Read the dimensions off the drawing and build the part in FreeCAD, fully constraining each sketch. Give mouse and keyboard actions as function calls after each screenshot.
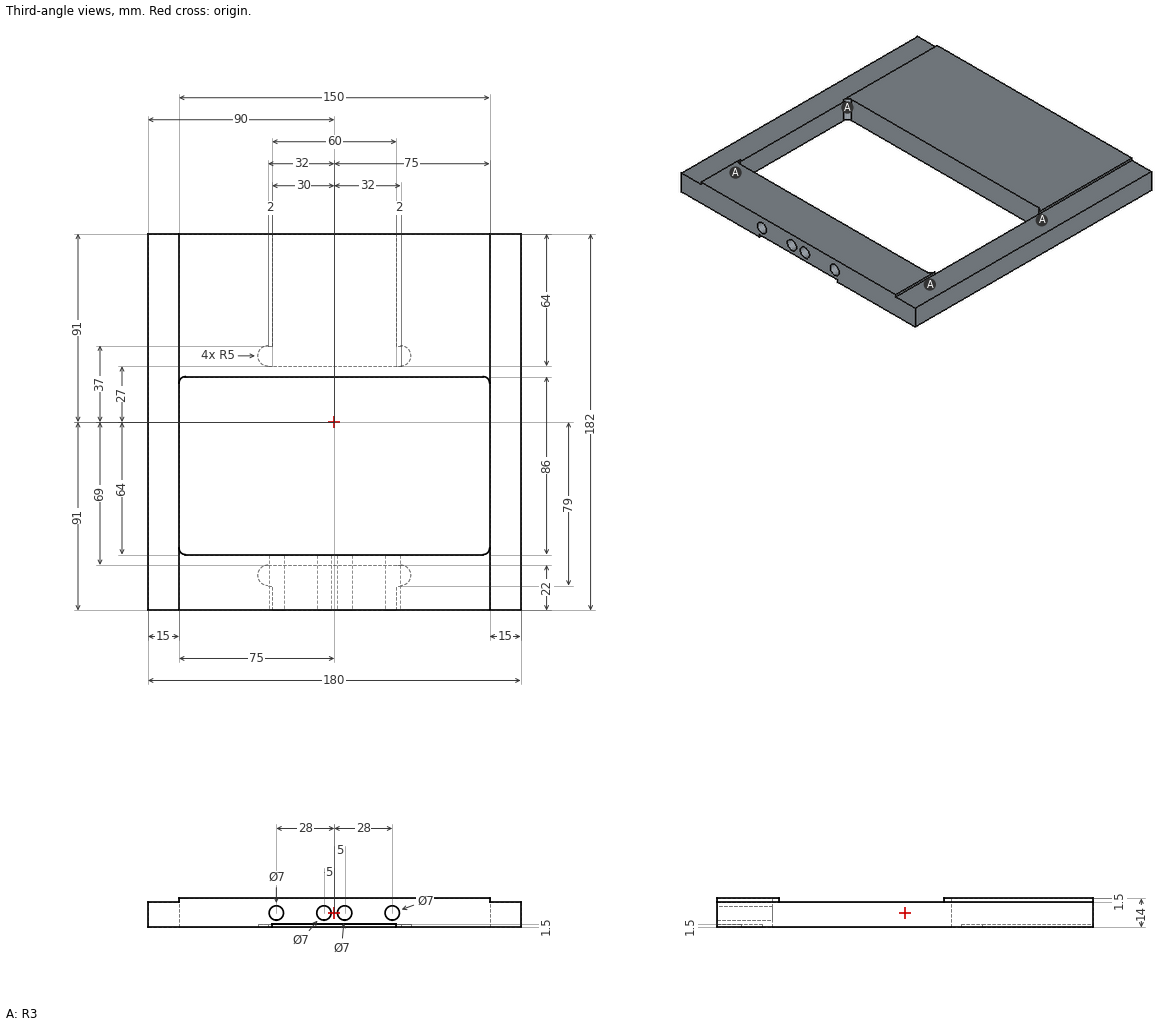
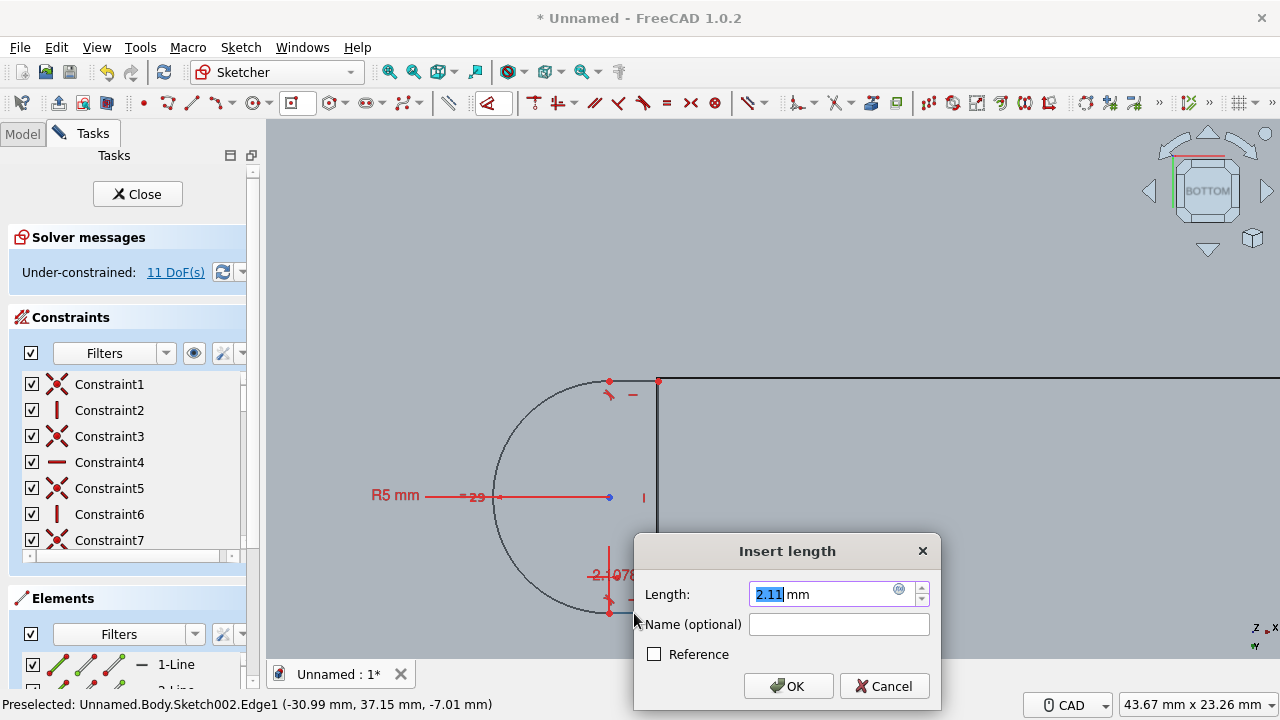
text(2)
key(Return)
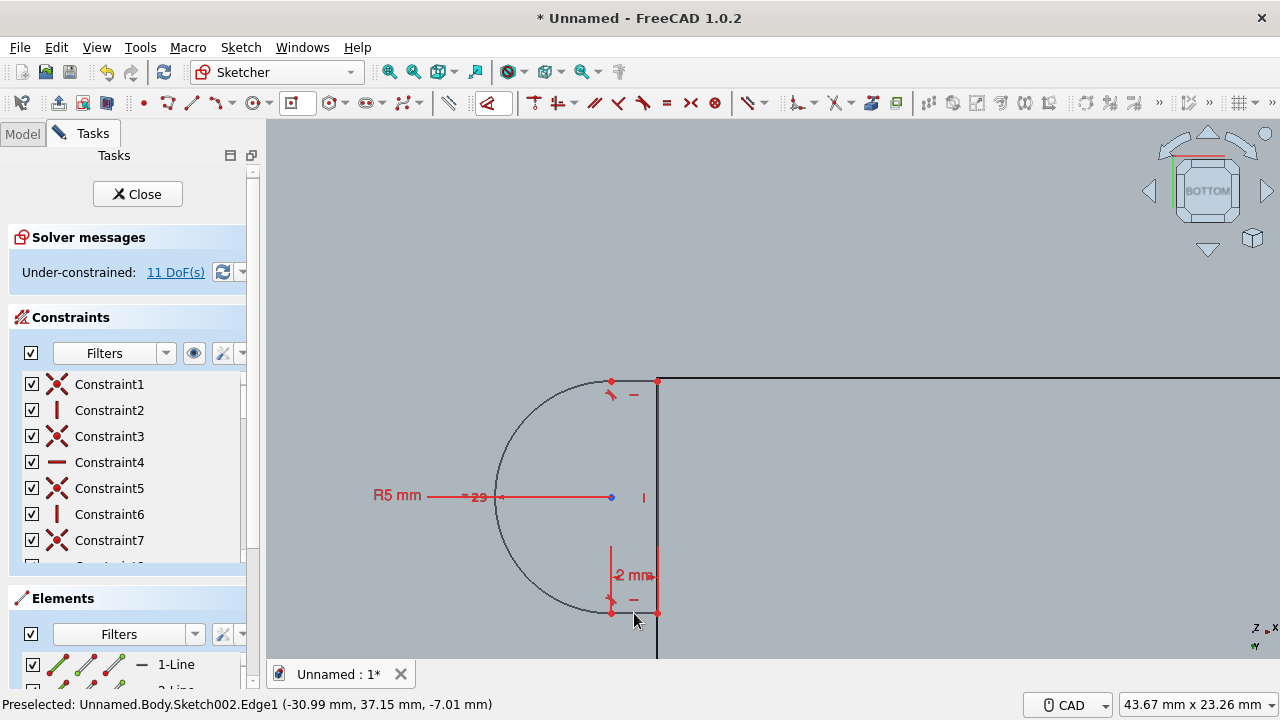
scroll(603, 565, down, 10)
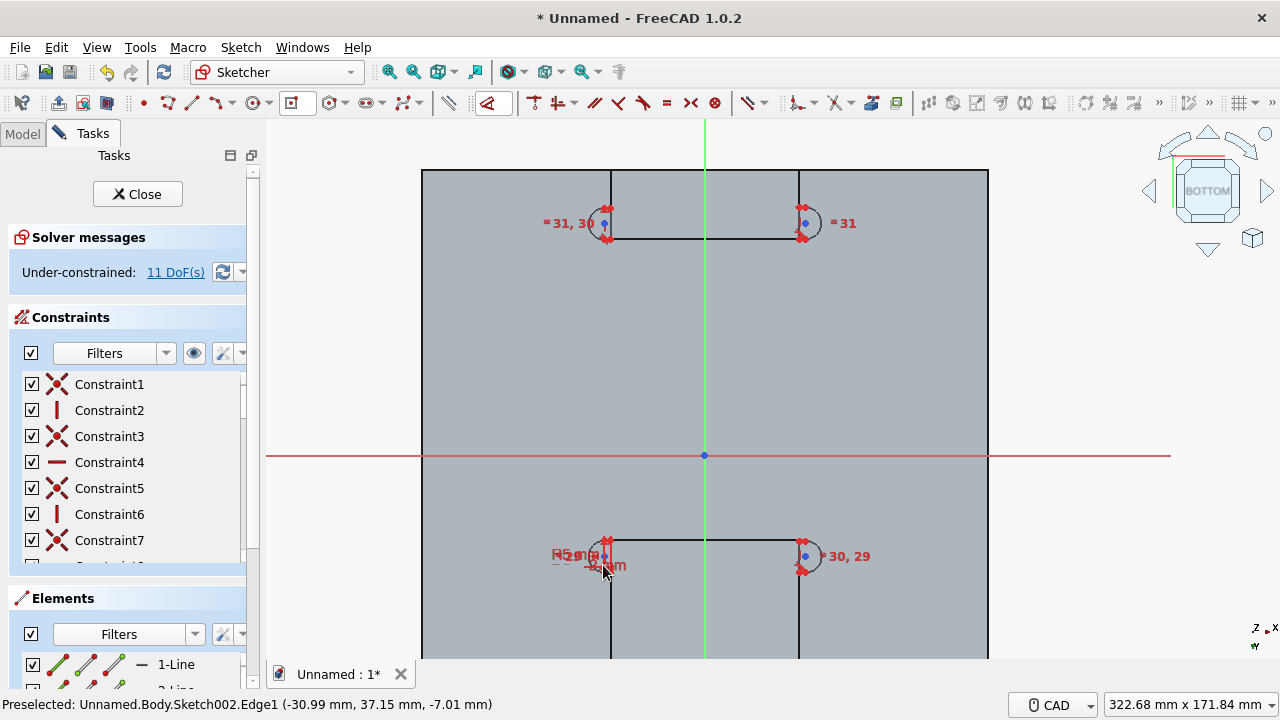
scroll(804, 541, up, 10)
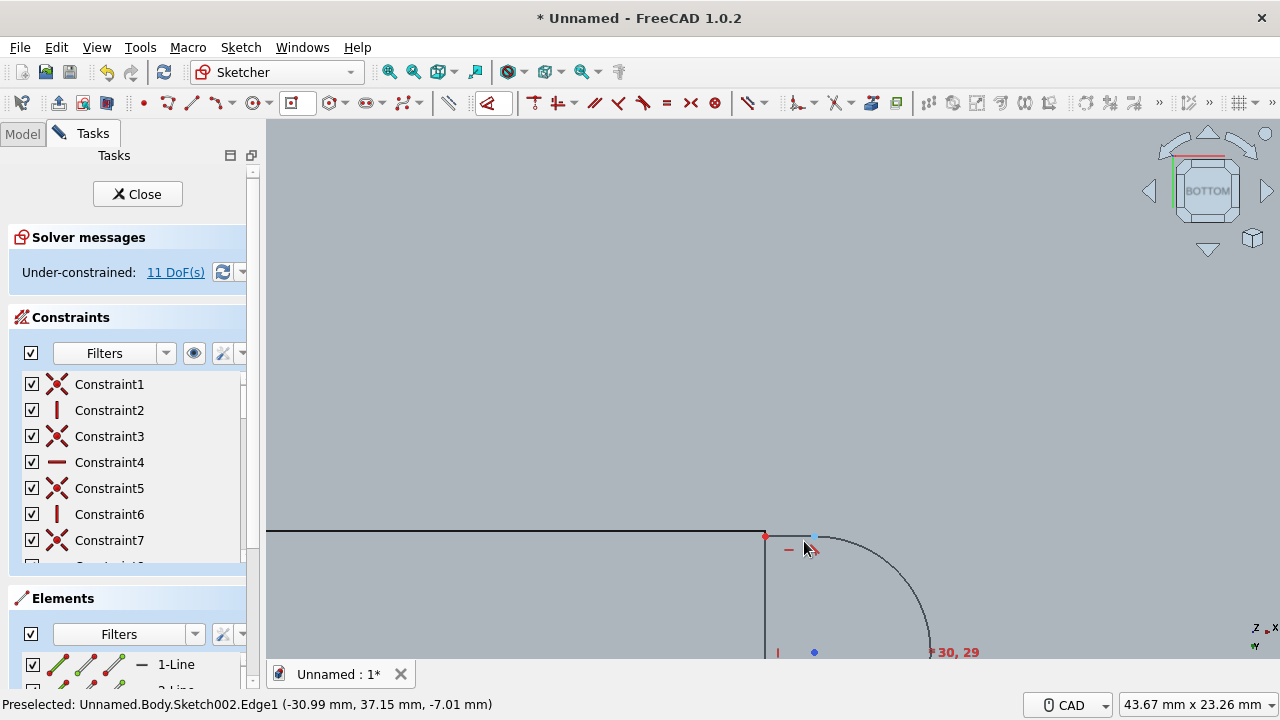
click(800, 536)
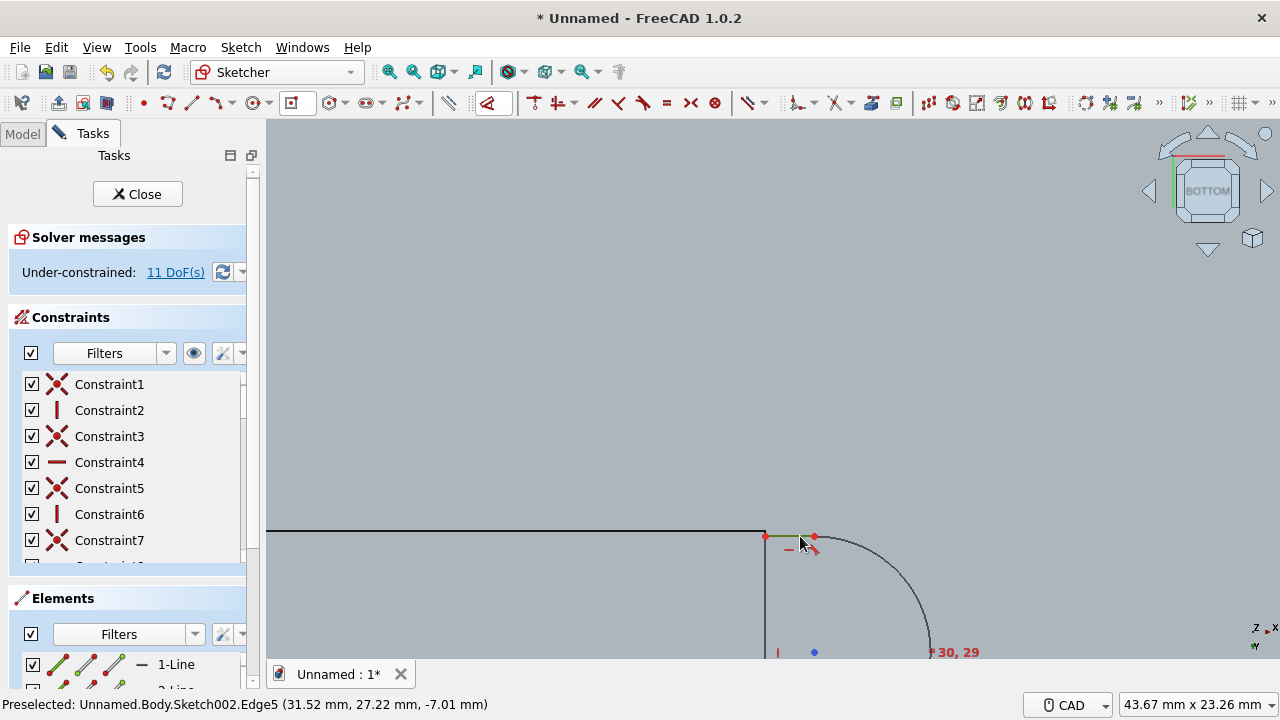
key(l)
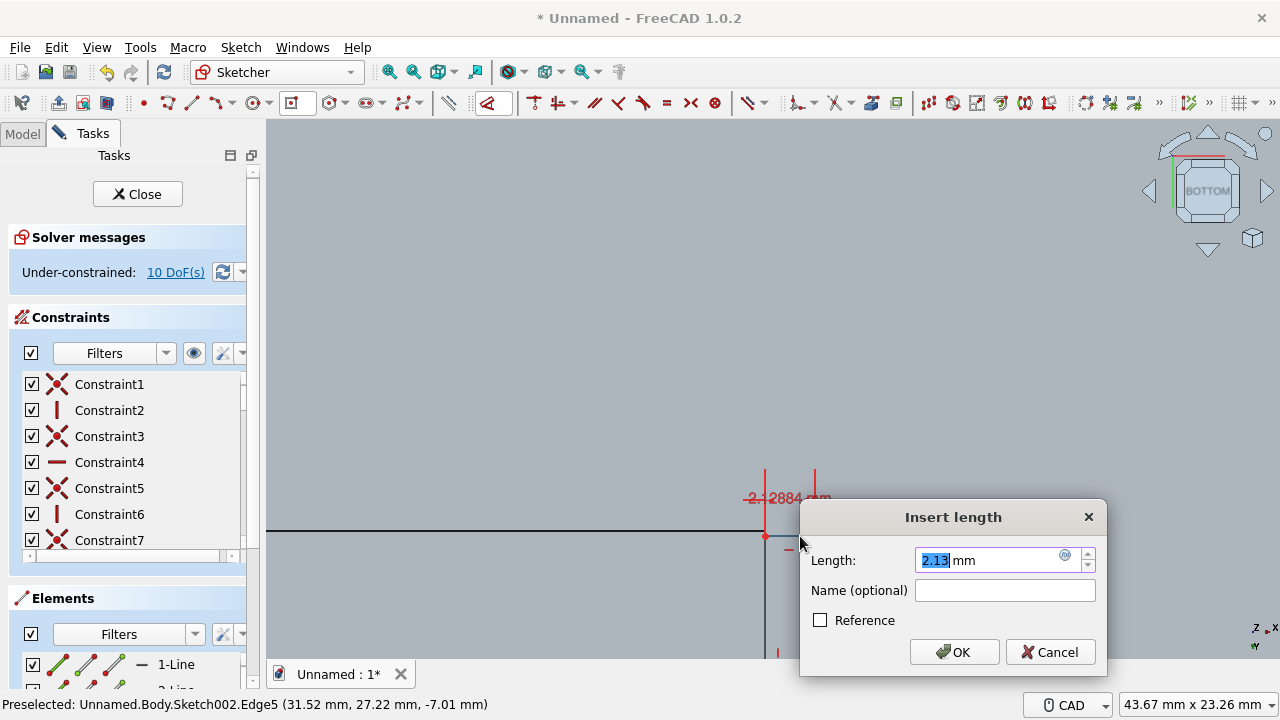
text(2)
key(Return)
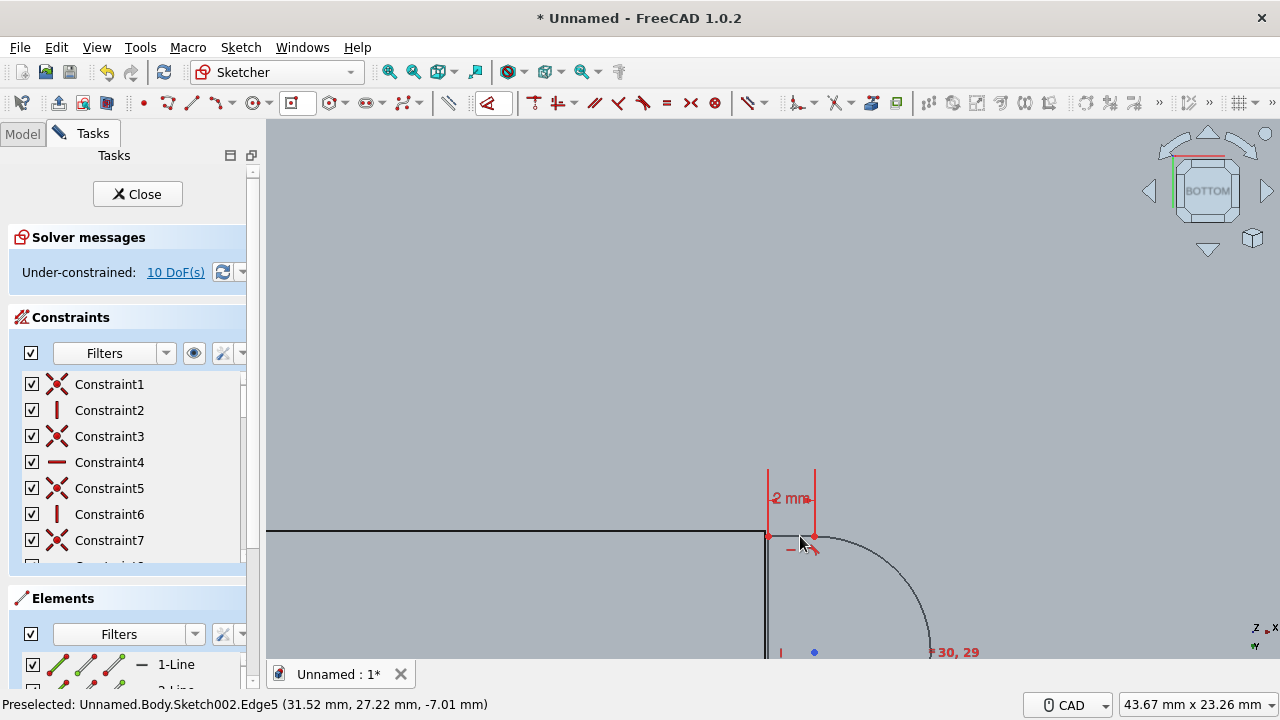
scroll(804, 541, down, 10)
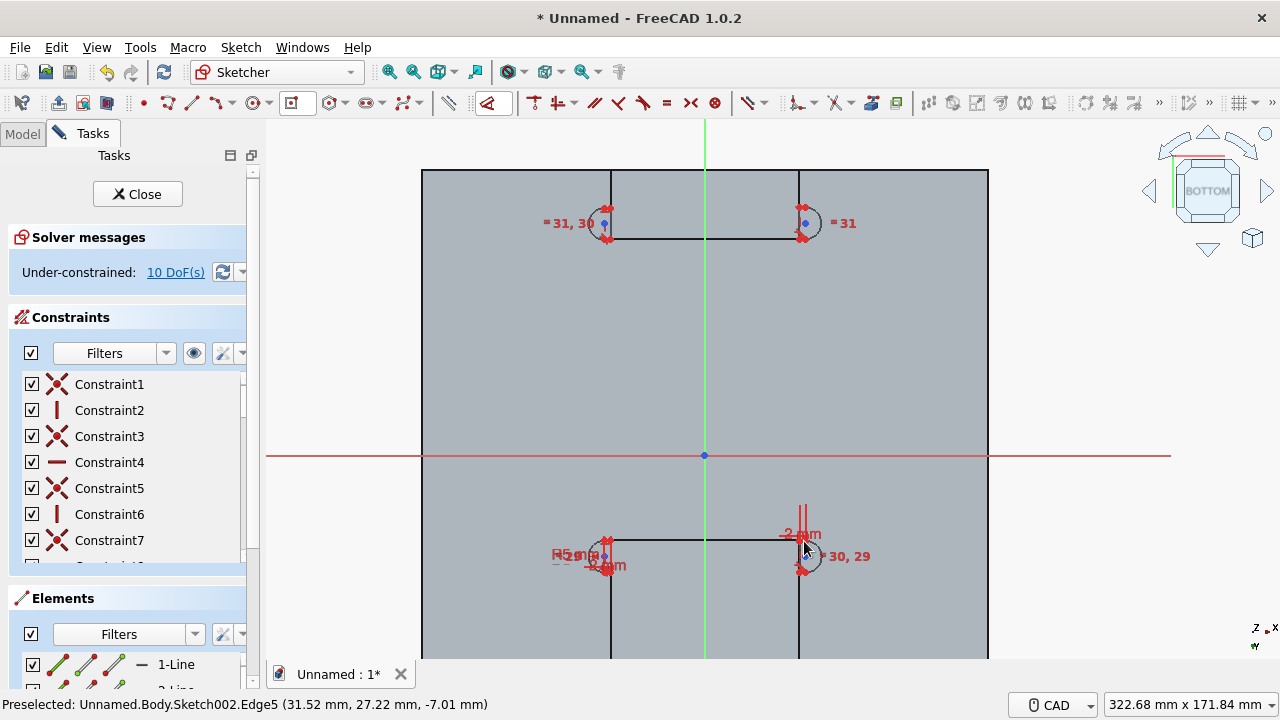
scroll(606, 240, up, 10)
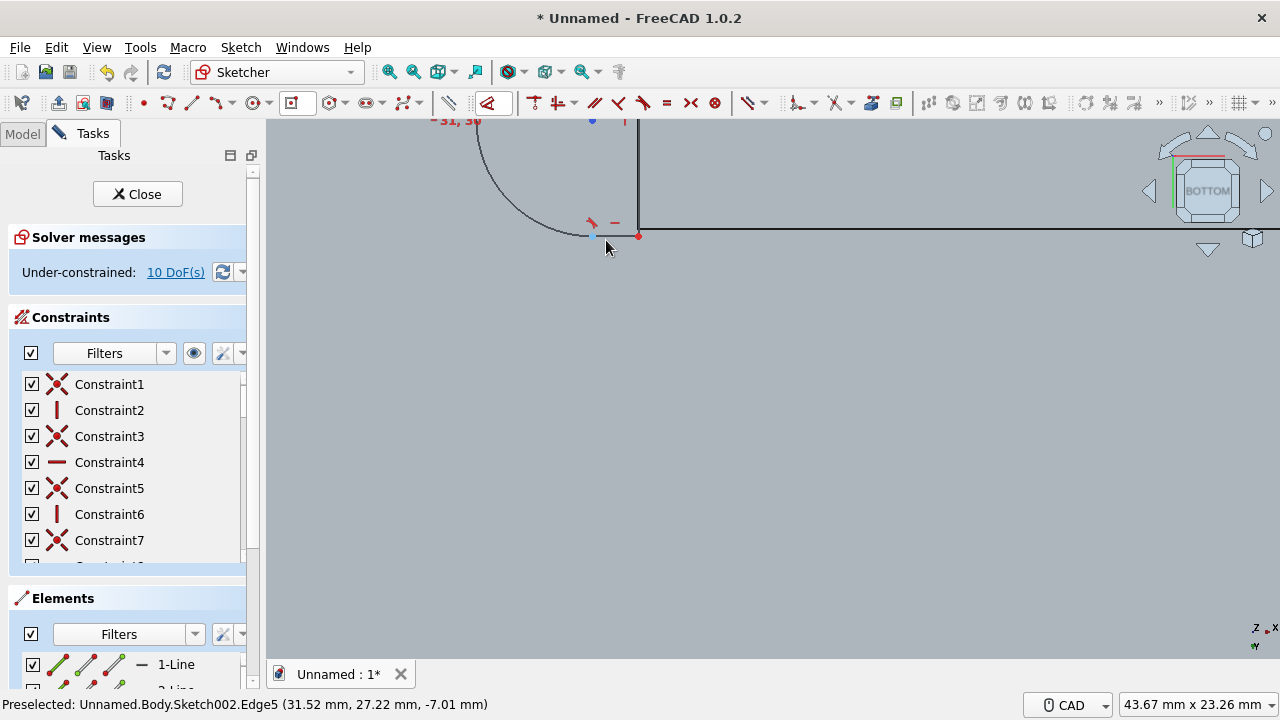
click(606, 236)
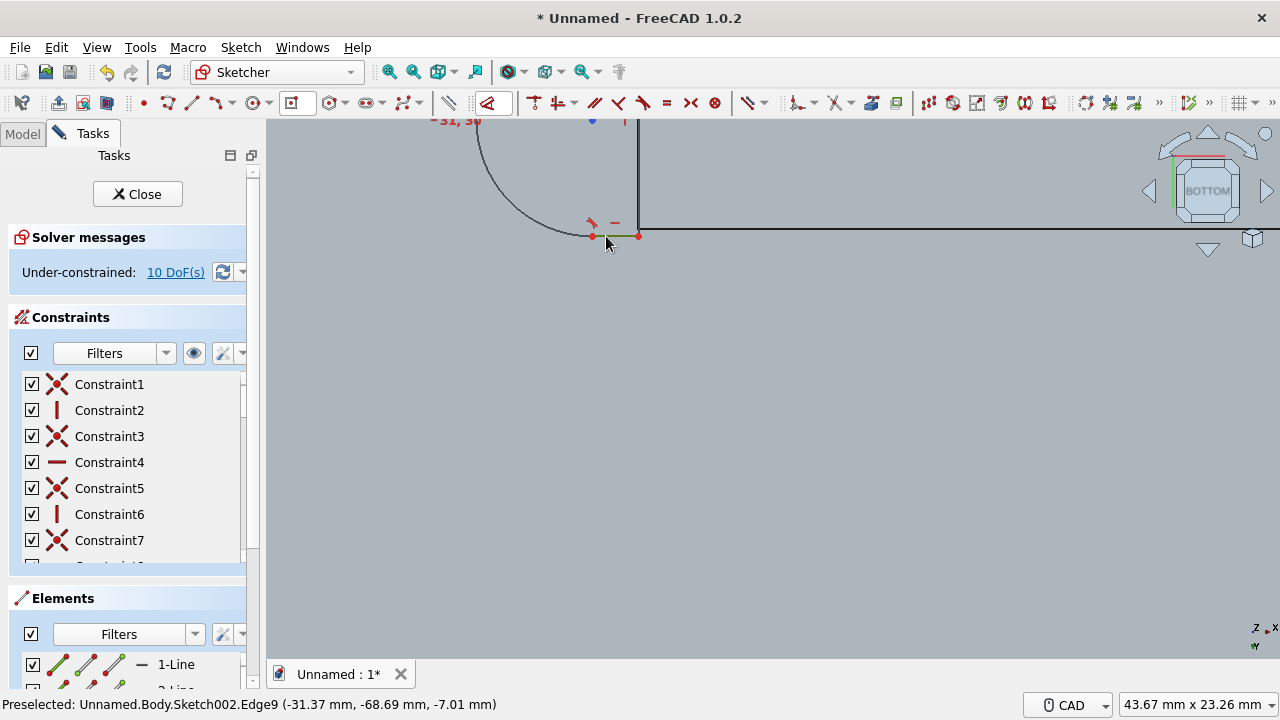
key(l)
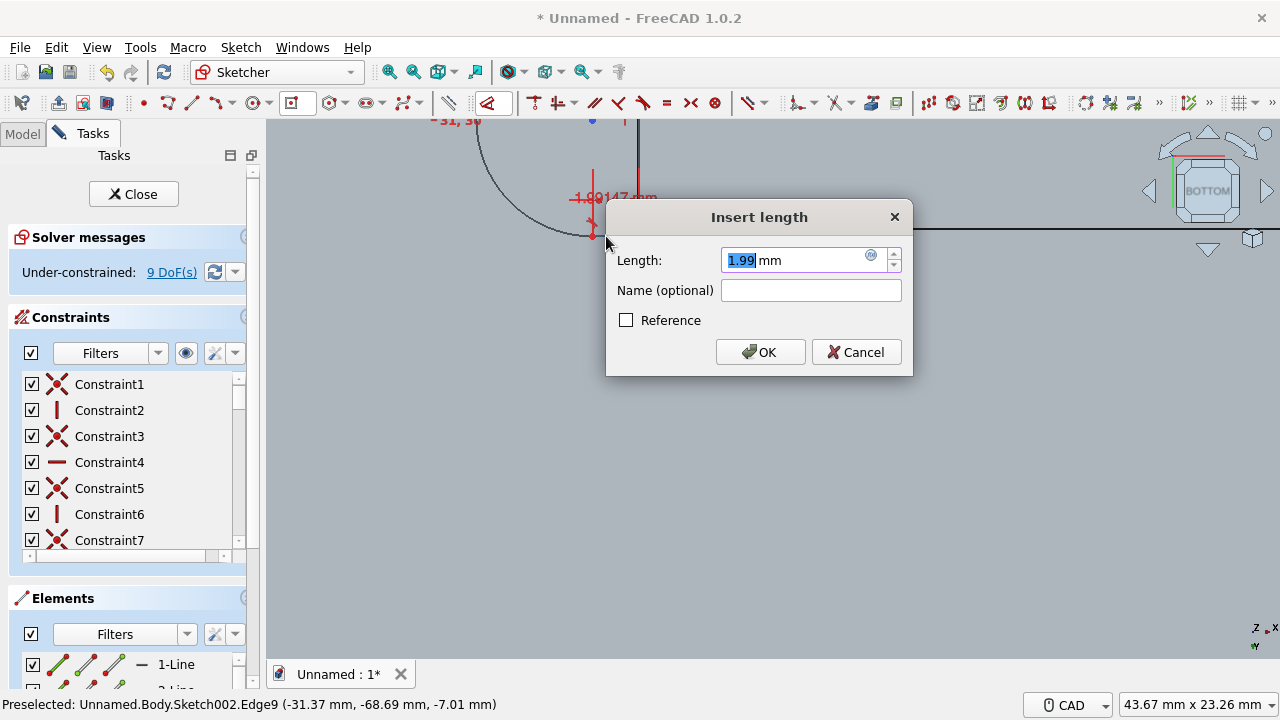
text(2)
key(Return)